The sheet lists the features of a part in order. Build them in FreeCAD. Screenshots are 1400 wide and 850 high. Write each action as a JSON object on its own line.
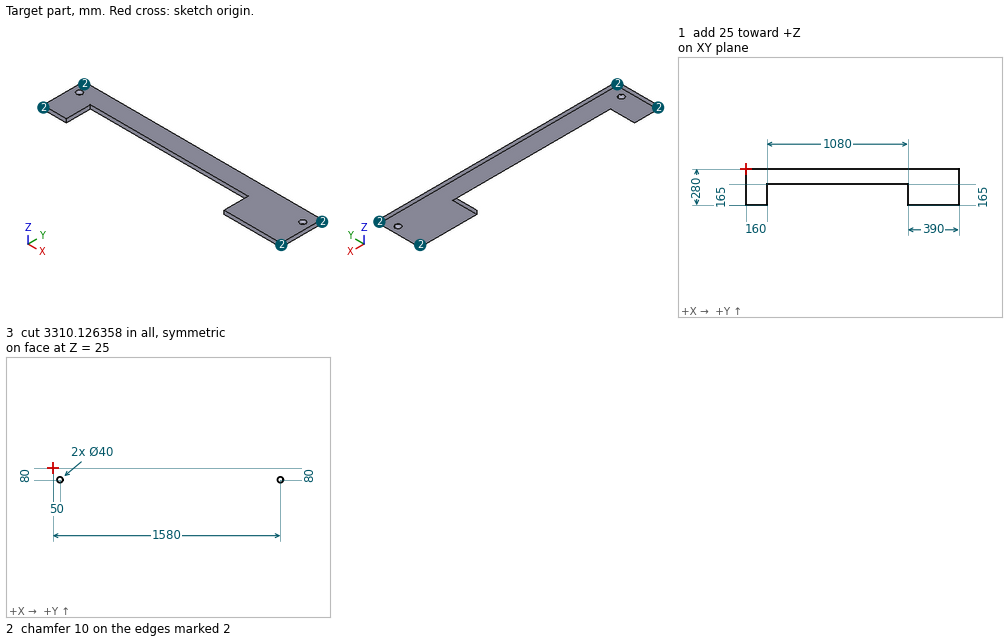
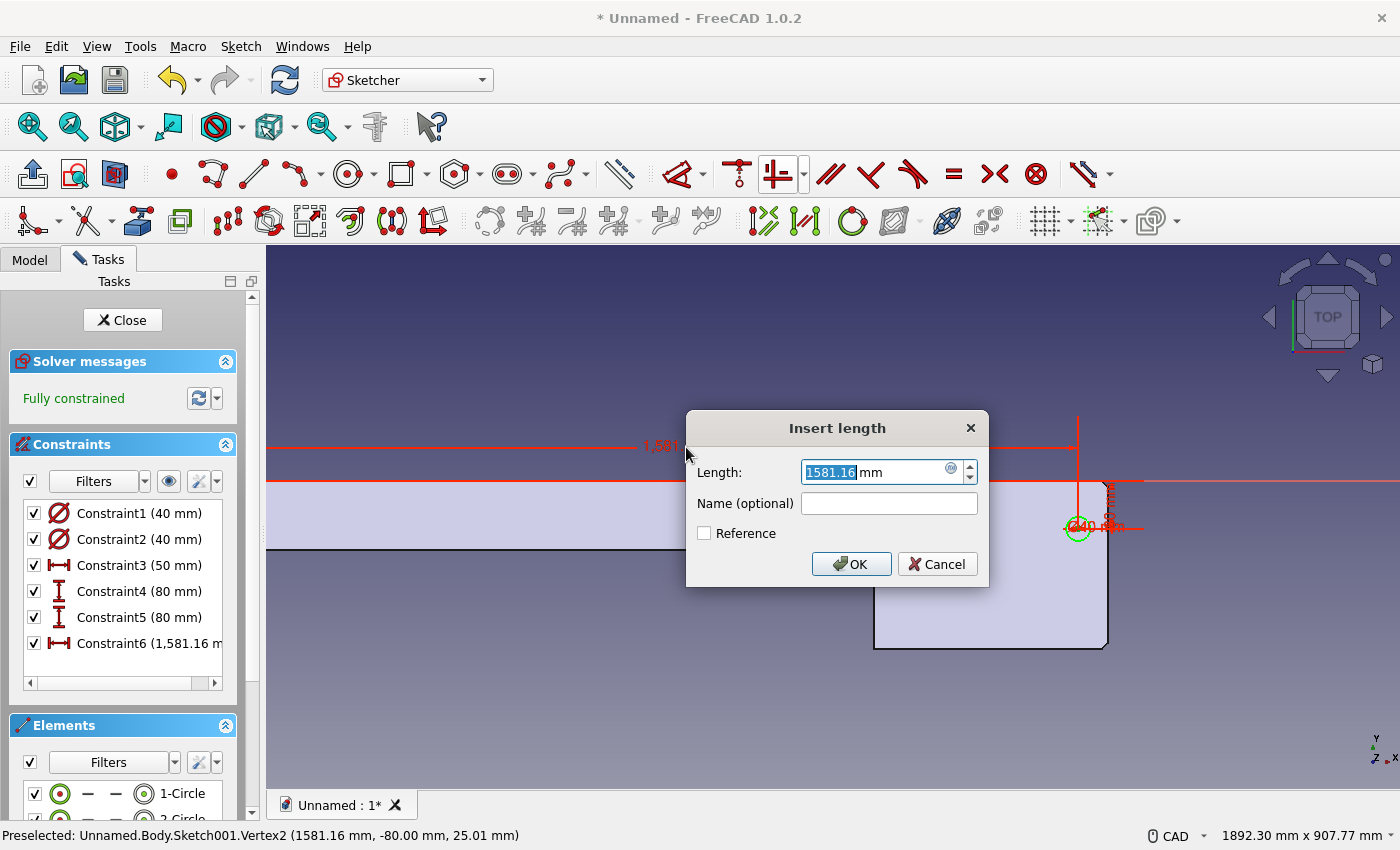
{"action": "type", "text": "1580"}
{"action": "key", "text": "Return"}
{"action": "key", "text": "Escape"}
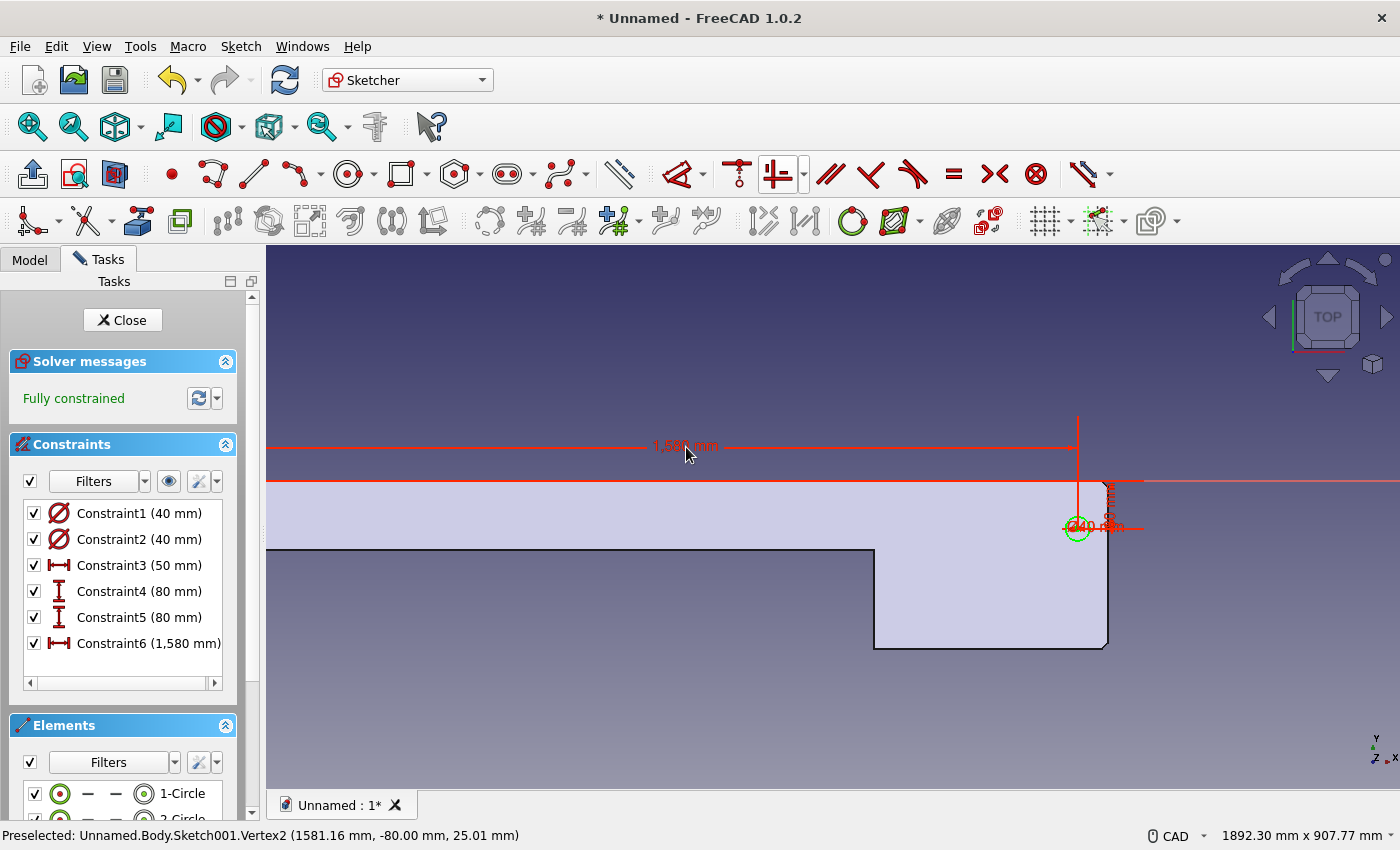
{"action": "left_click", "coordinate": [123, 320]}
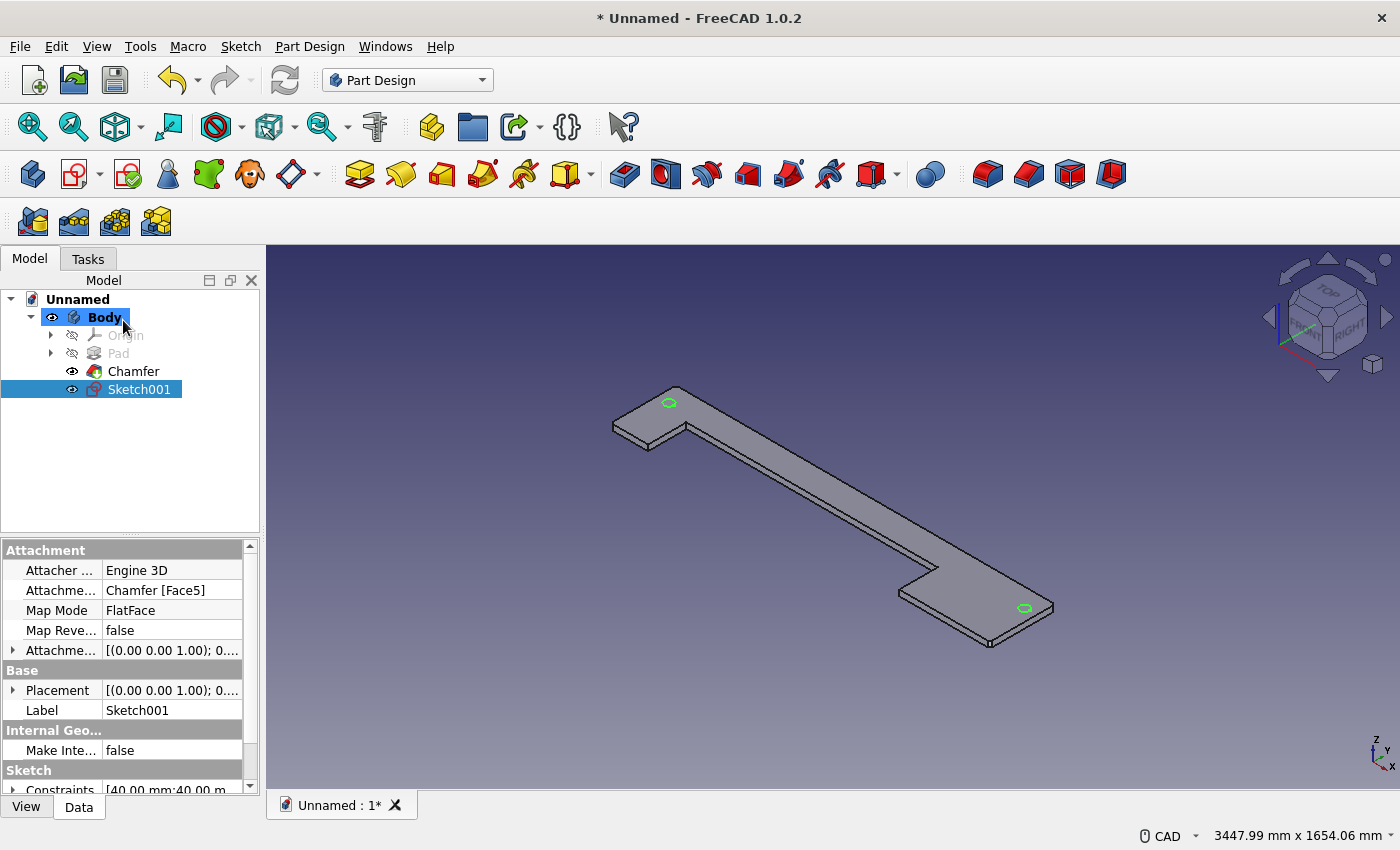
{"action": "left_click", "coordinate": [625, 174]}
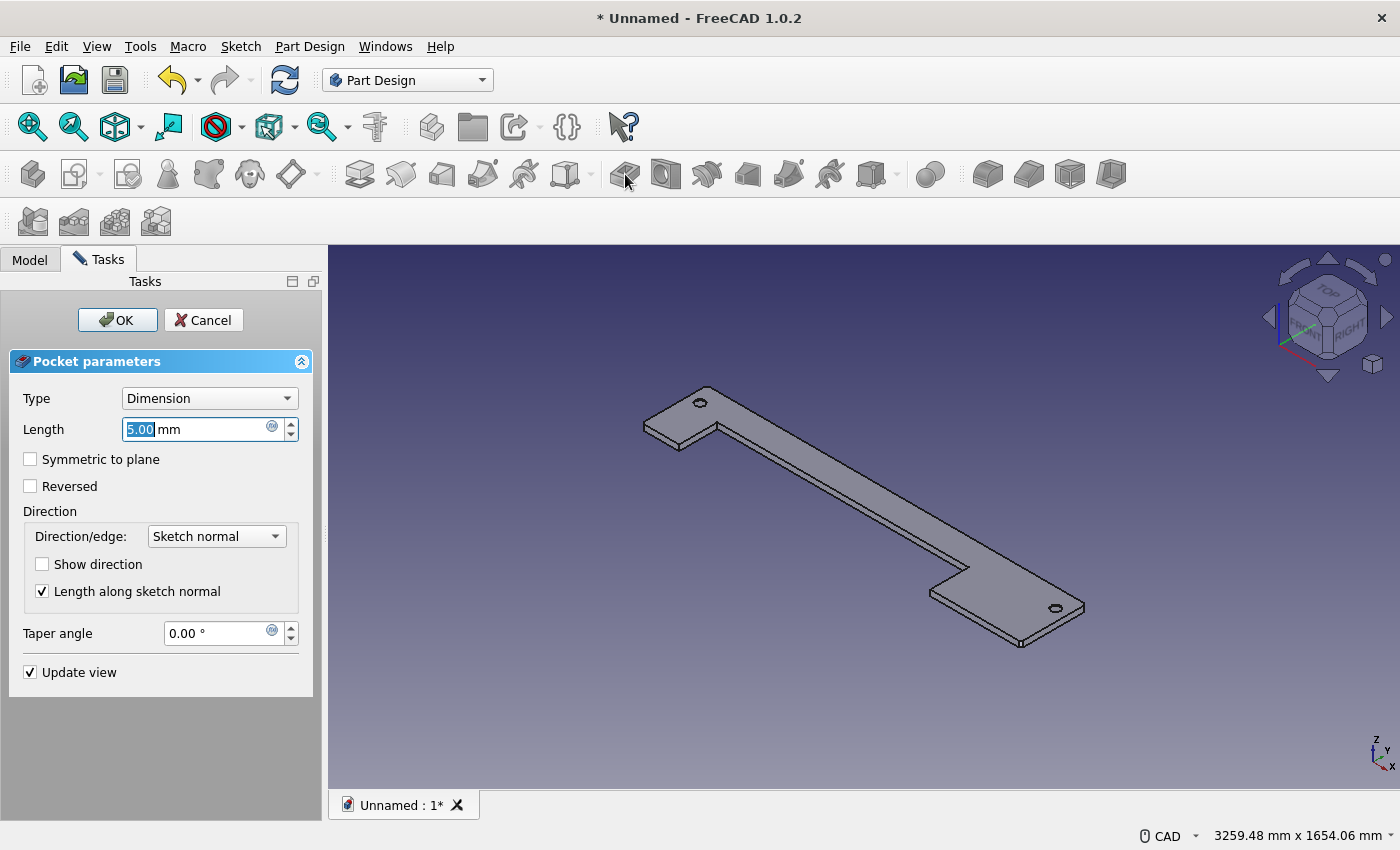
{"action": "type", "text": "3310.126358"}
{"action": "key", "text": "Tab"}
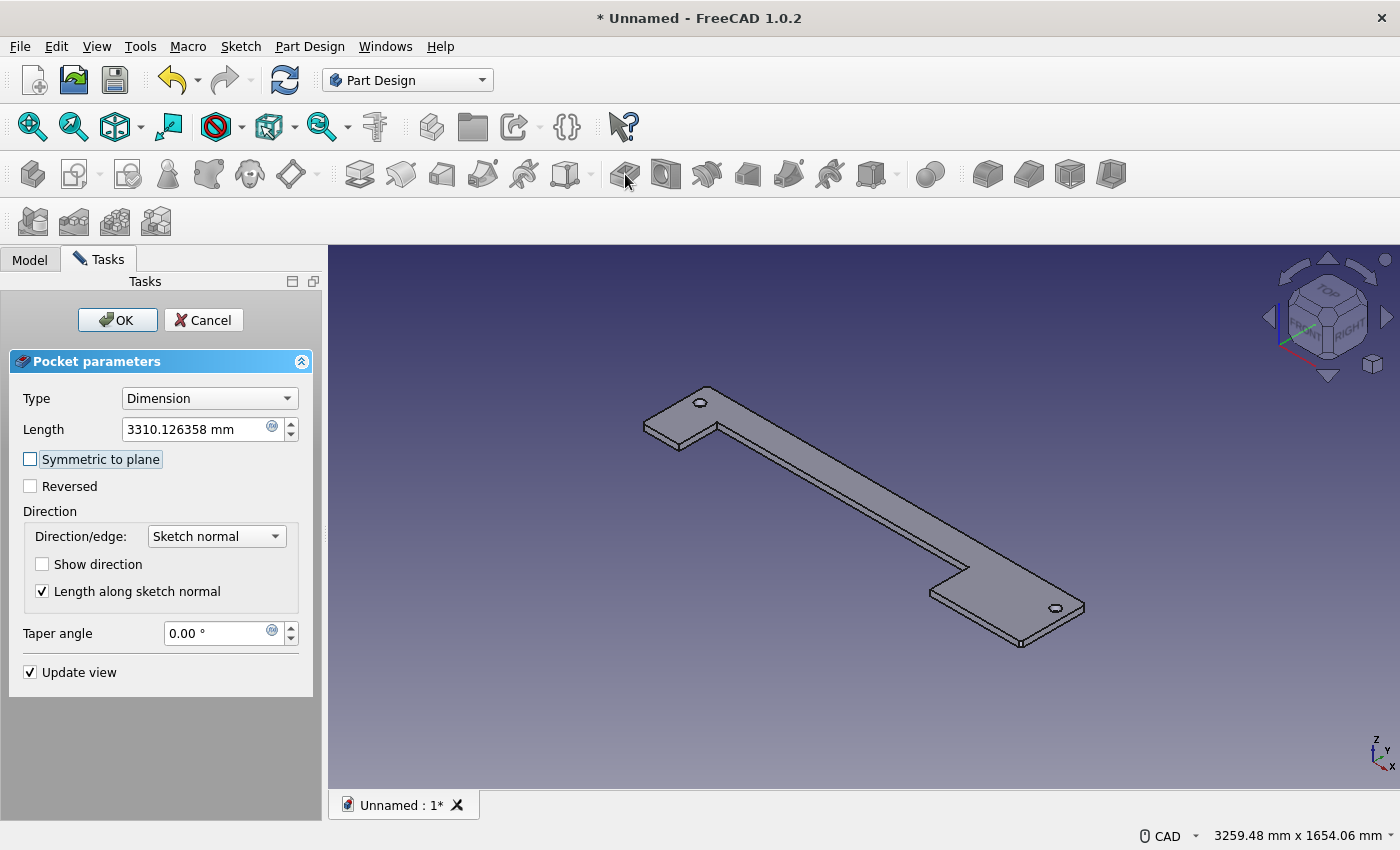
{"action": "left_click", "coordinate": [31, 459]}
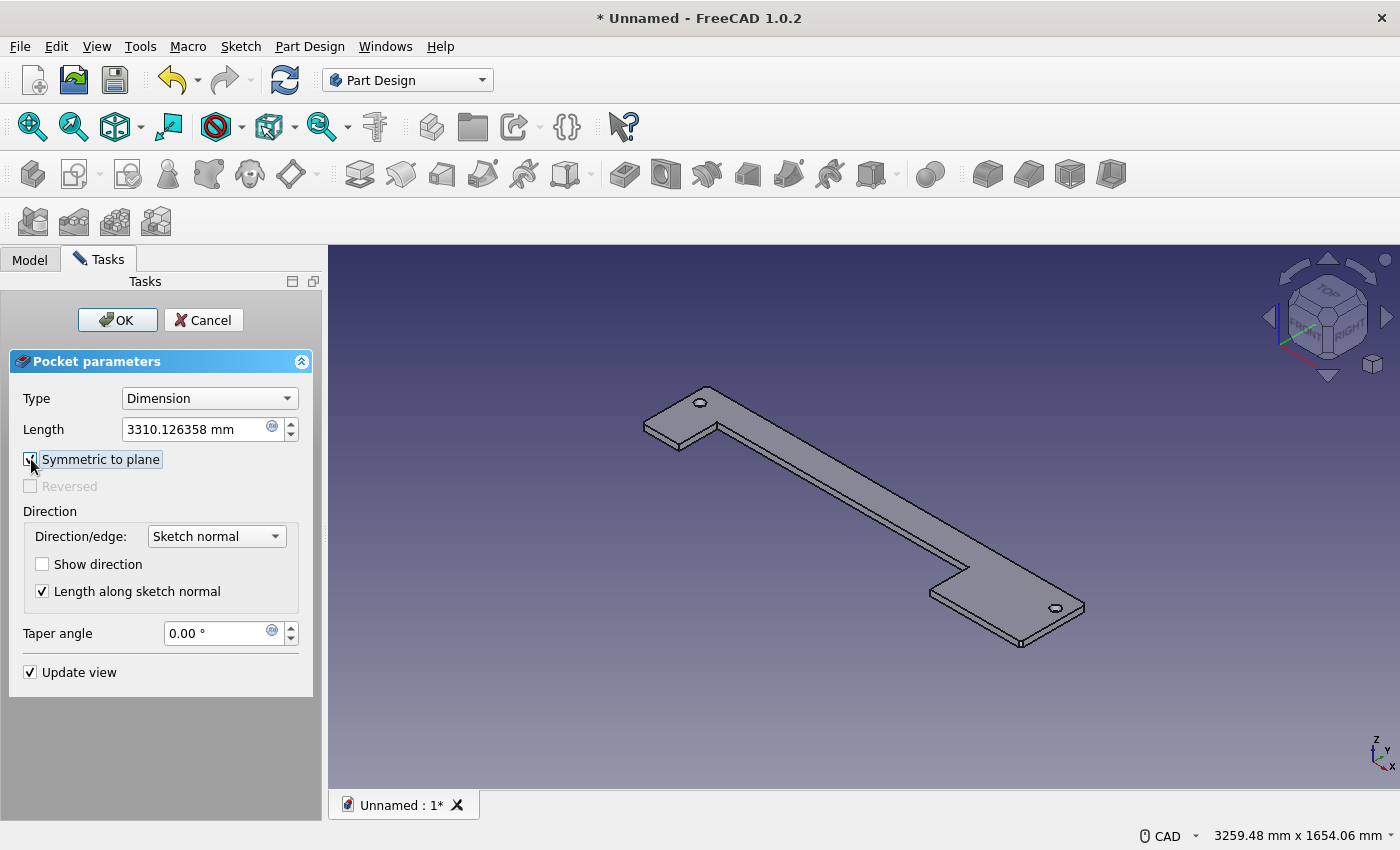
{"action": "left_click", "coordinate": [118, 320]}